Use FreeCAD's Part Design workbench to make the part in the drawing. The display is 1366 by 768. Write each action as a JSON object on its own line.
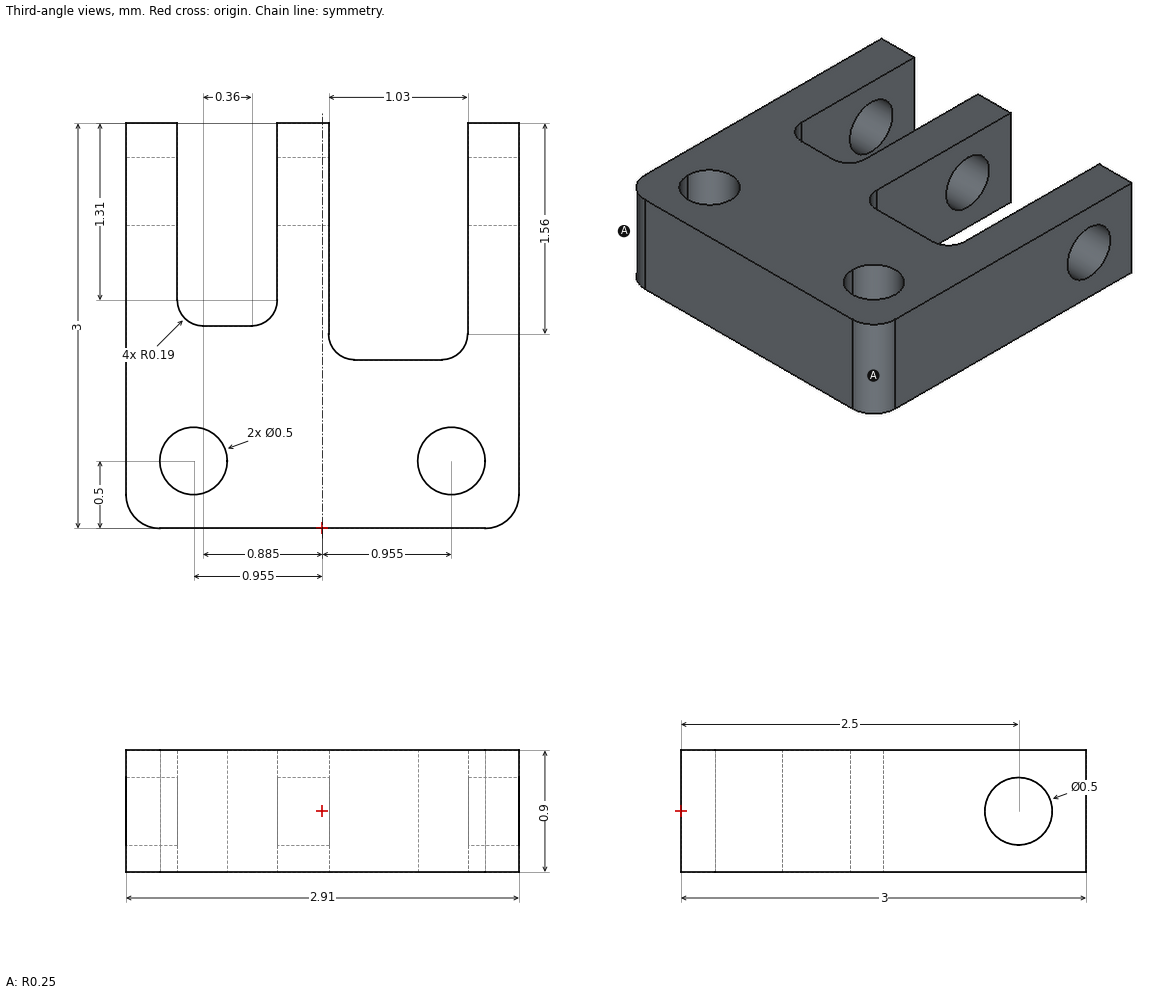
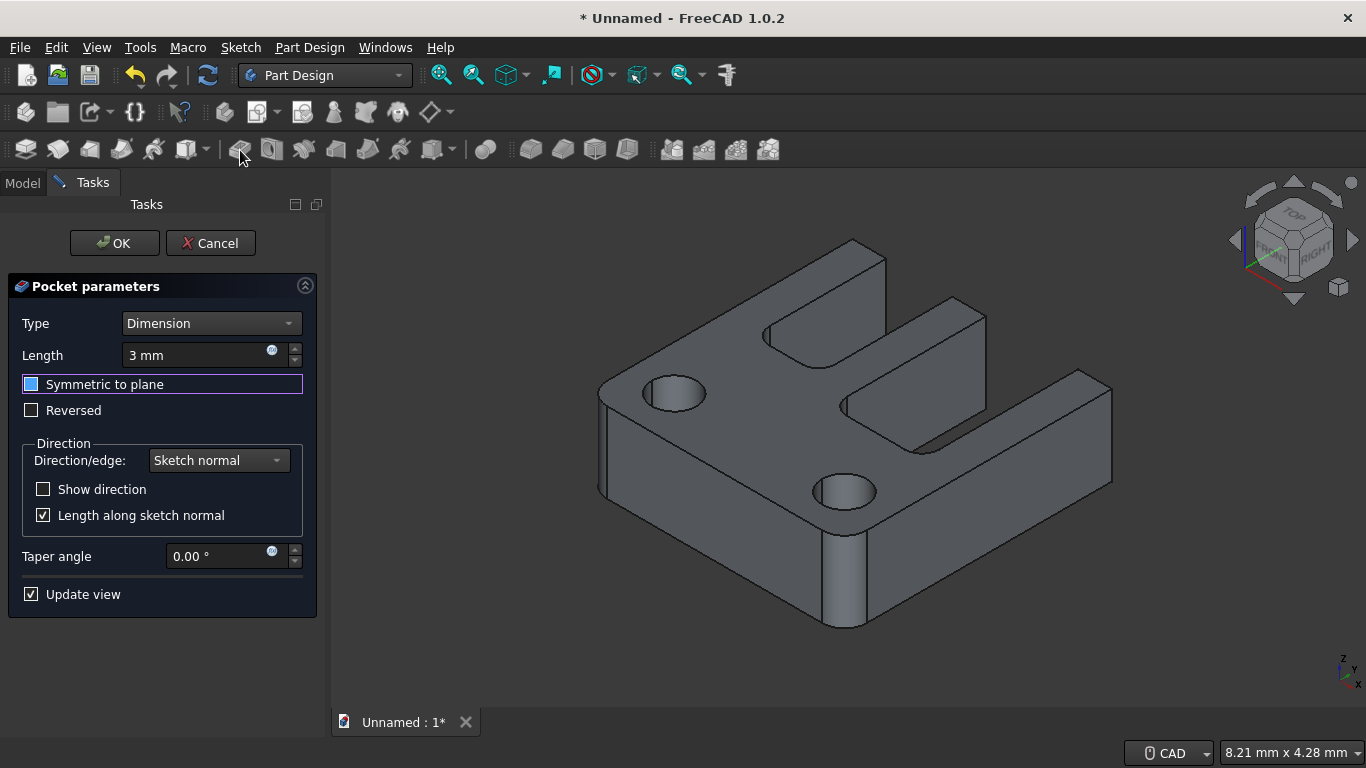
{"action": "left_click", "coordinate": [115, 243]}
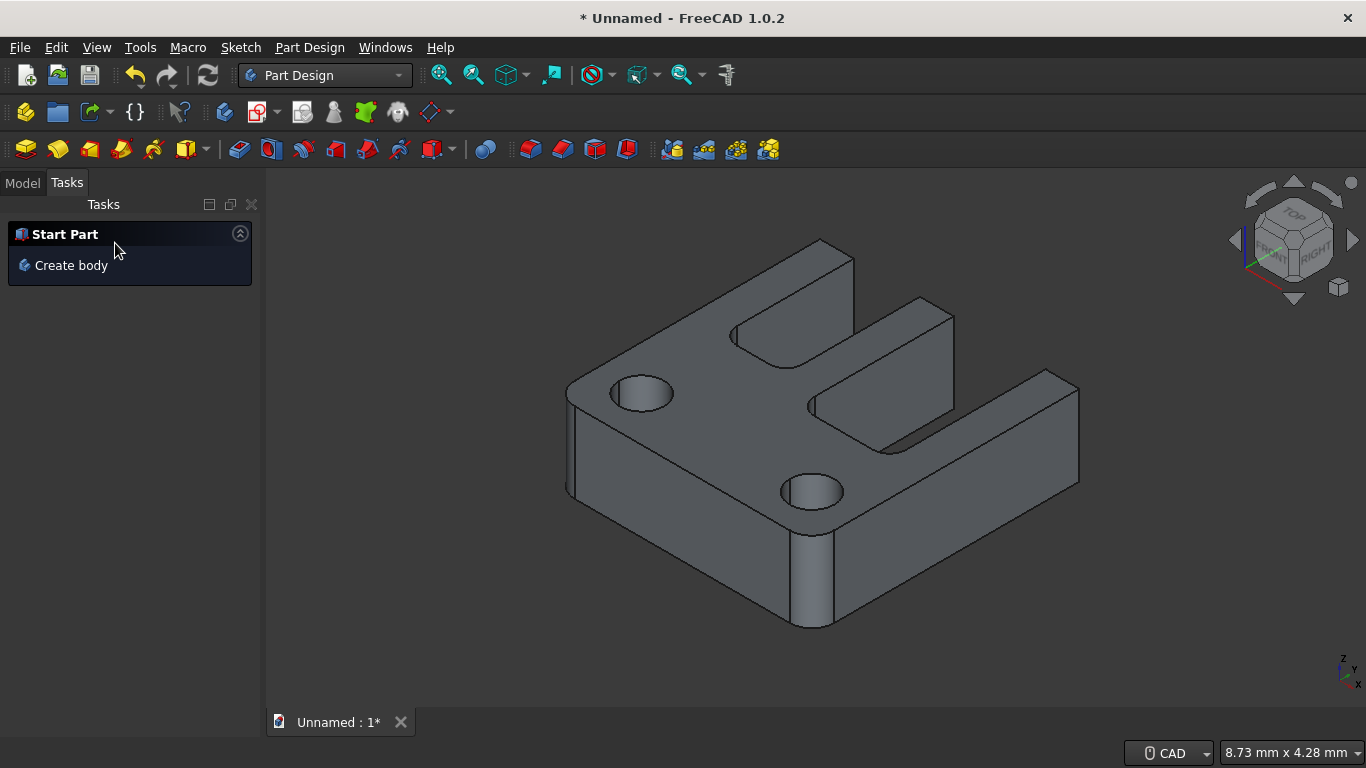
{"action": "left_click", "coordinate": [992, 485]}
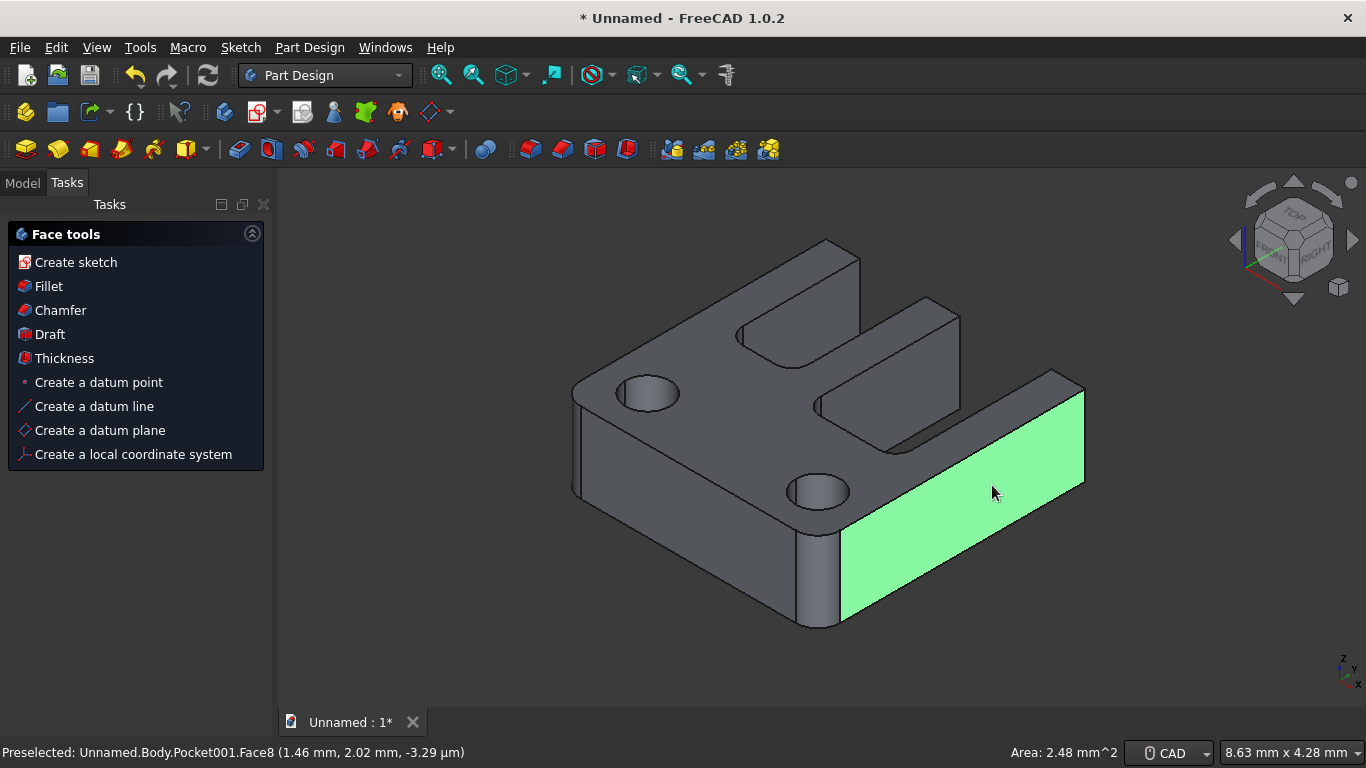
{"action": "left_click", "coordinate": [258, 112]}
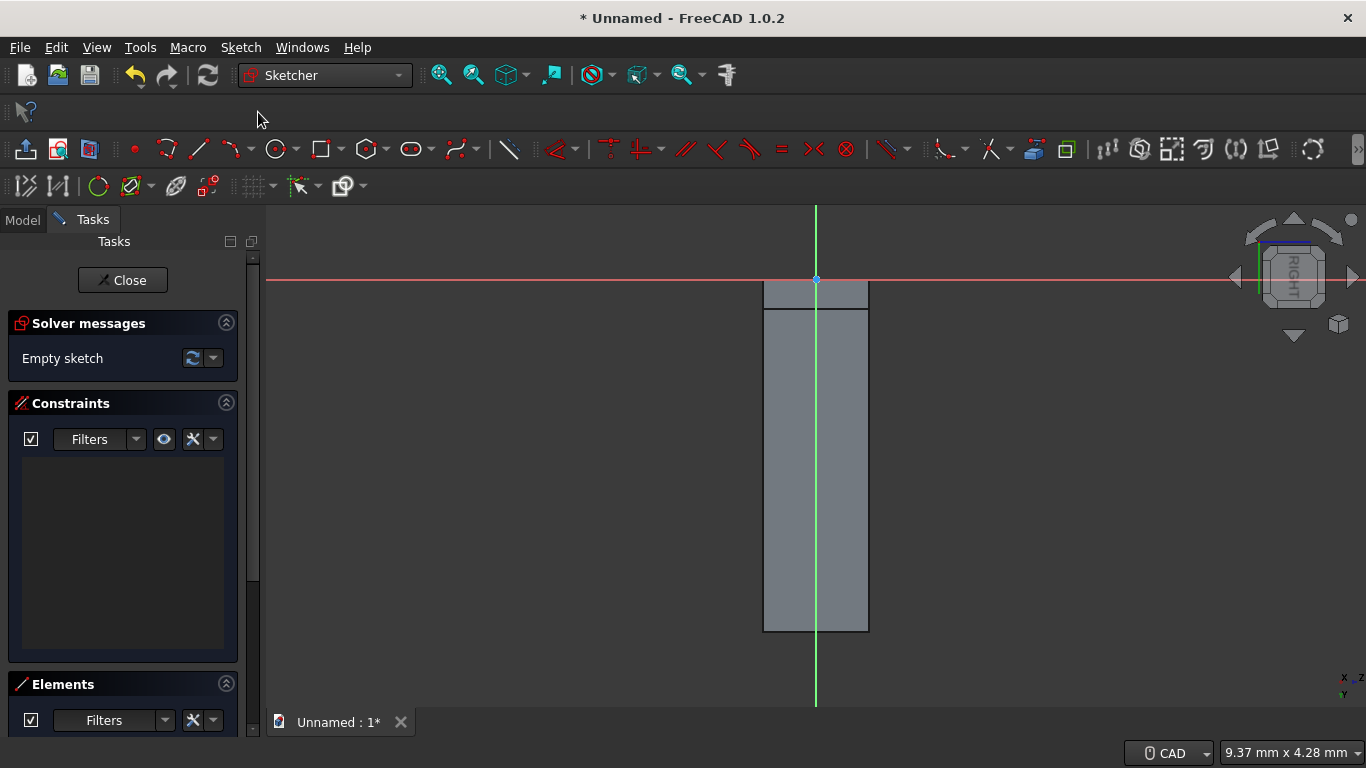
{"action": "scroll", "coordinate": [833, 603], "scroll_direction": "up", "scroll_amount": 8}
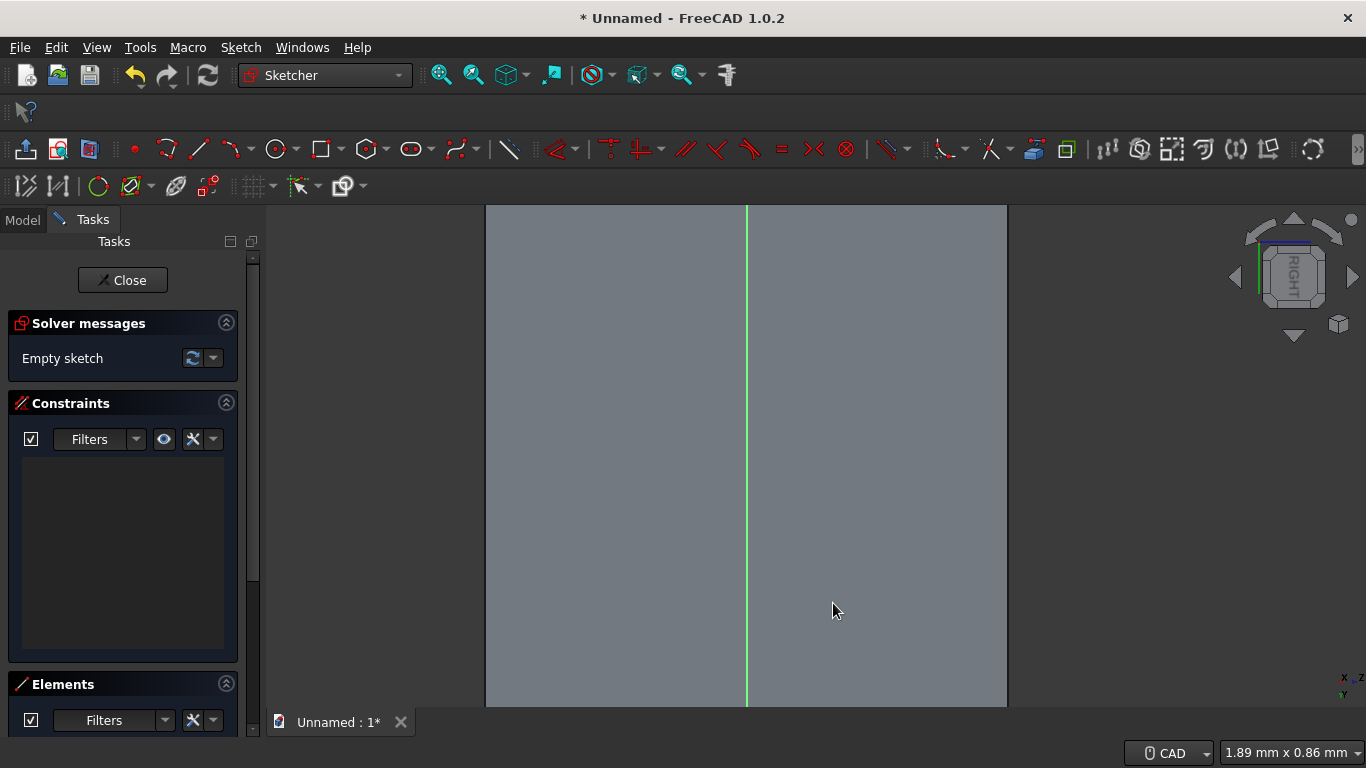
{"action": "left_click", "coordinate": [276, 150]}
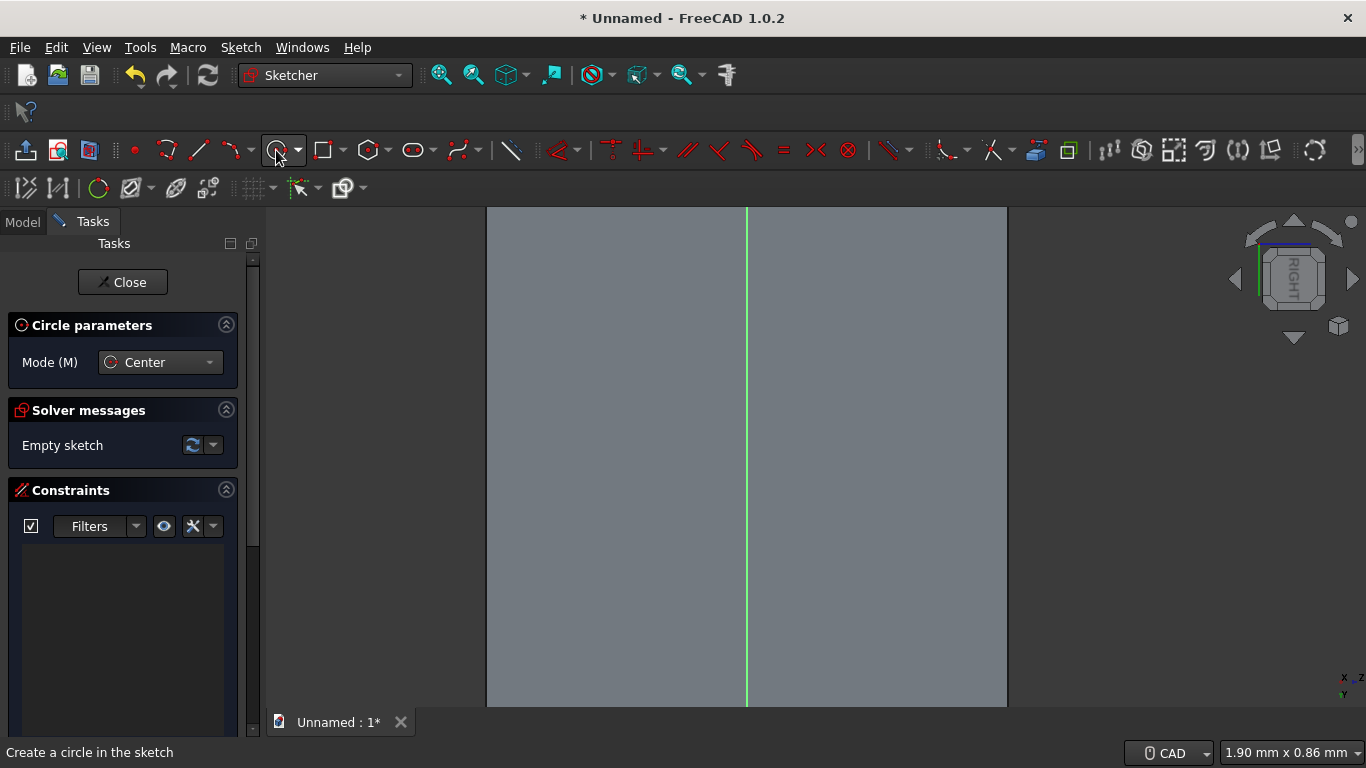
{"action": "left_click", "coordinate": [747, 454]}
{"action": "left_click", "coordinate": [849, 352]}
{"action": "key", "text": "Escape"}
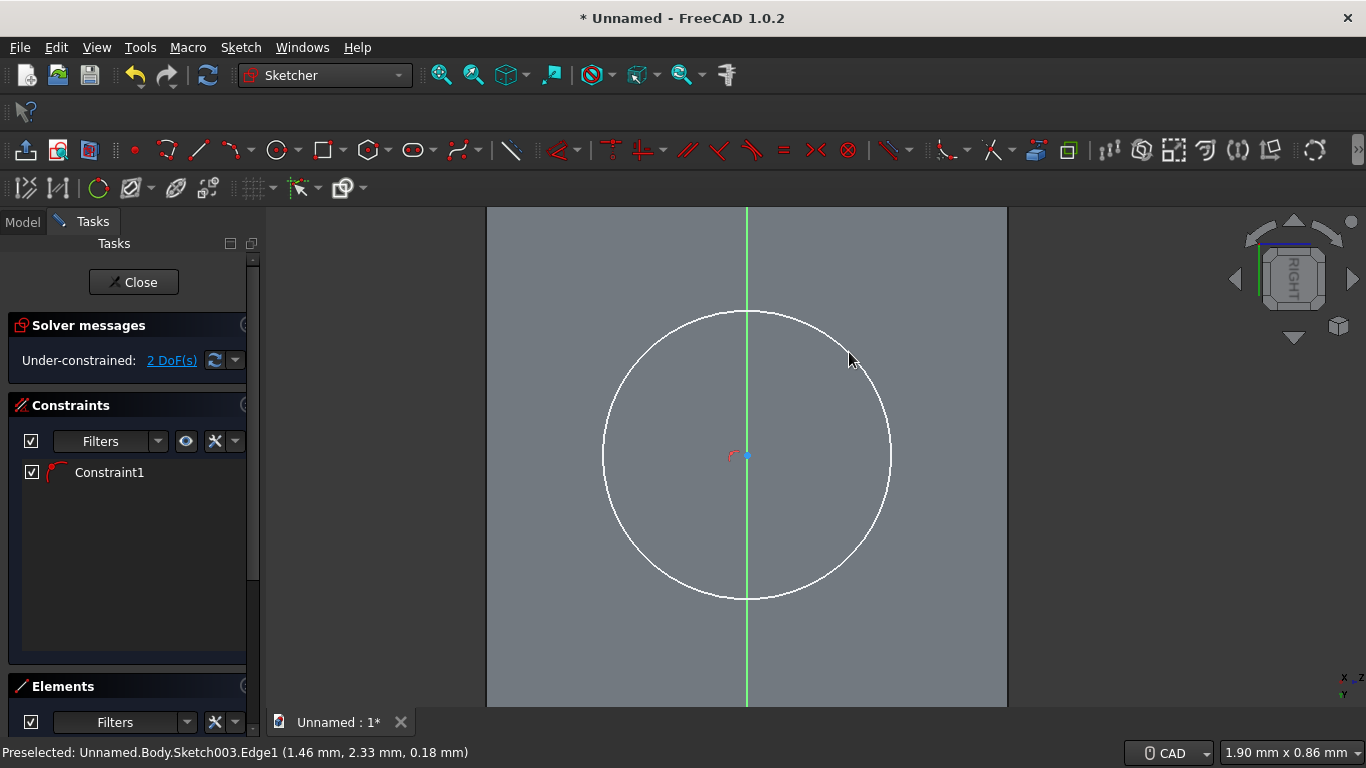
{"action": "key", "text": "d"}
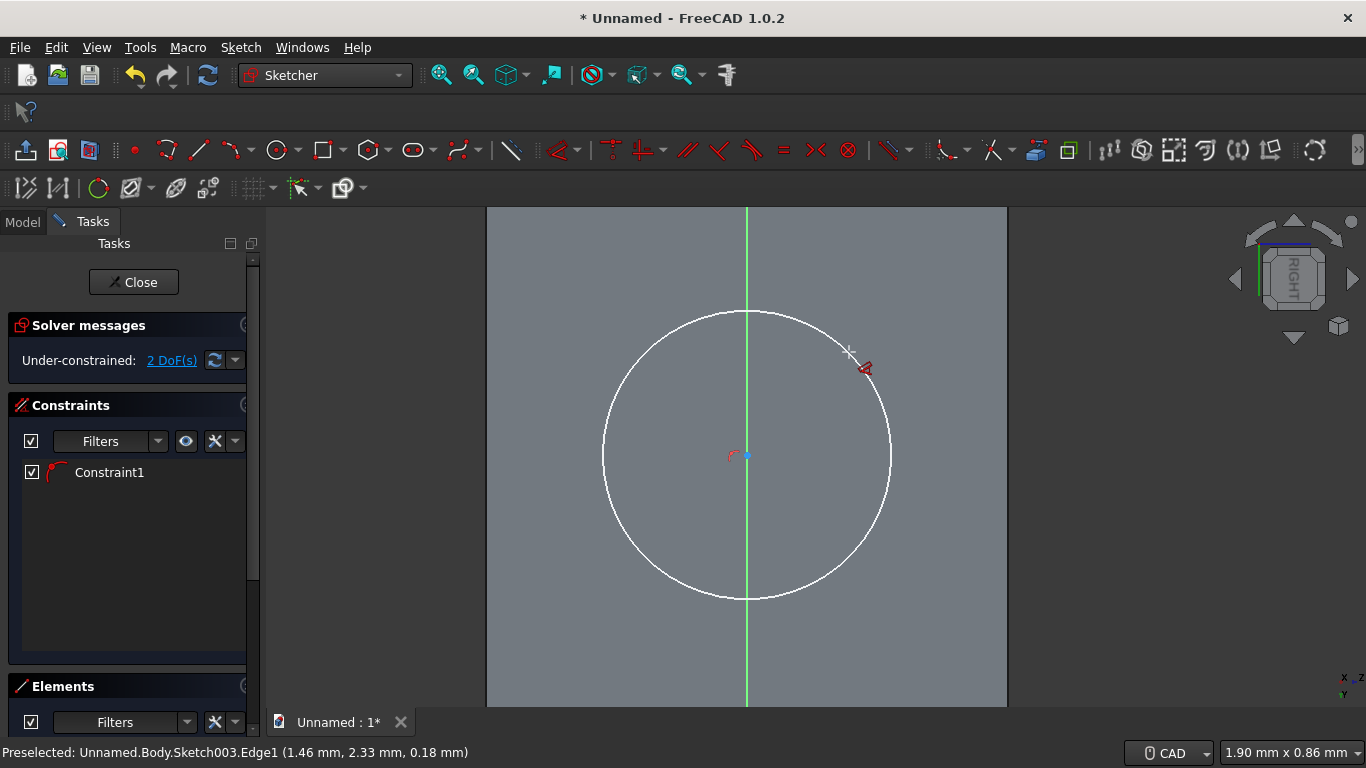
{"action": "left_click", "coordinate": [849, 353]}
{"action": "left_click", "coordinate": [872, 330]}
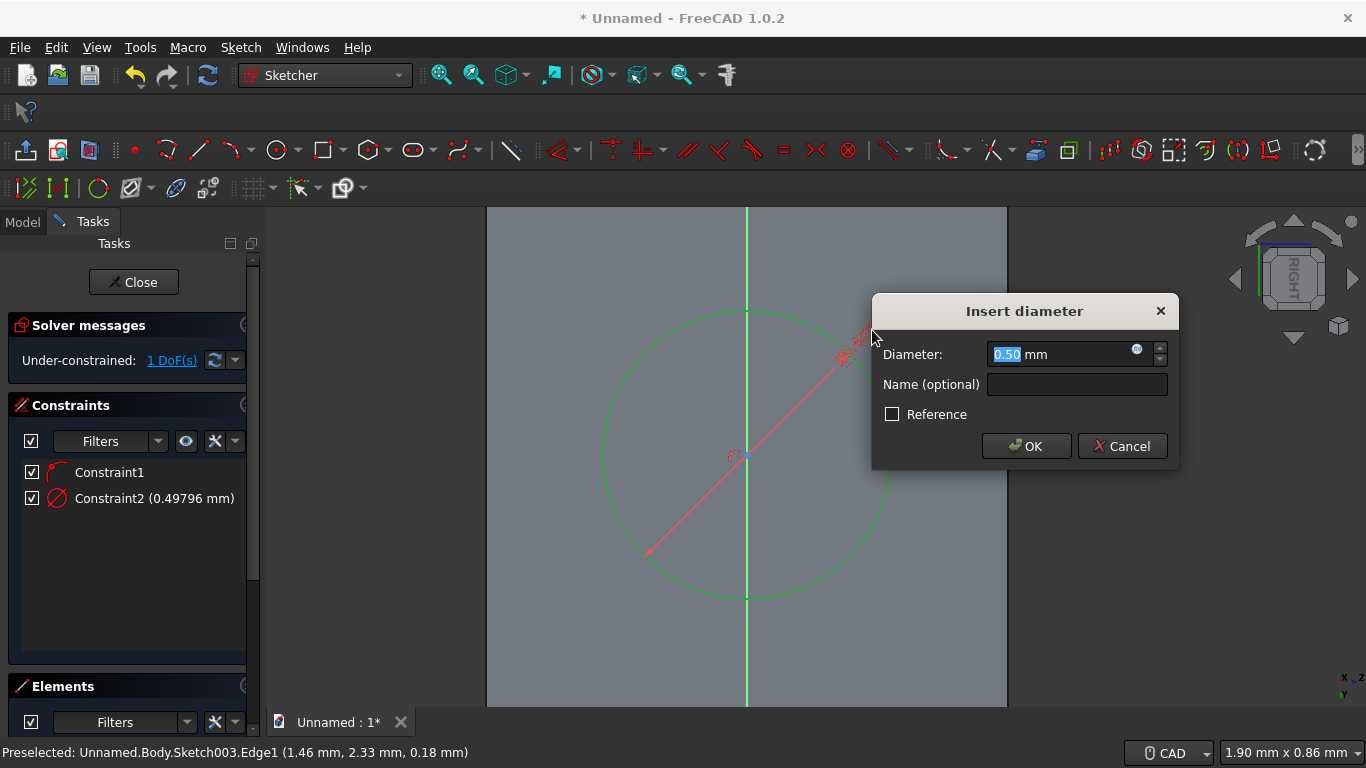
{"action": "type", "text": "0.5"}
{"action": "key", "text": "Return"}